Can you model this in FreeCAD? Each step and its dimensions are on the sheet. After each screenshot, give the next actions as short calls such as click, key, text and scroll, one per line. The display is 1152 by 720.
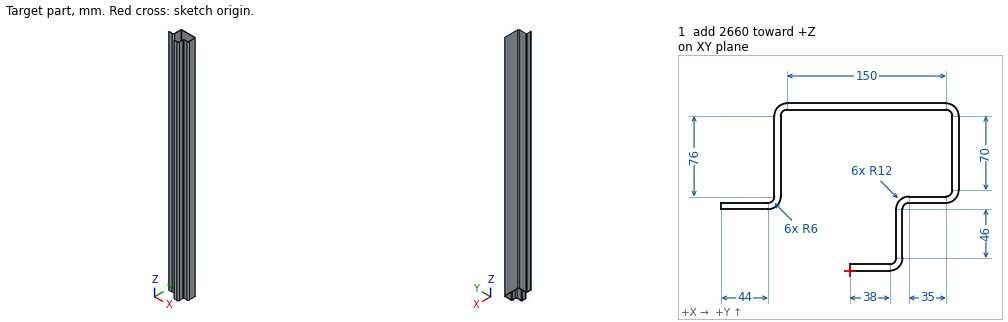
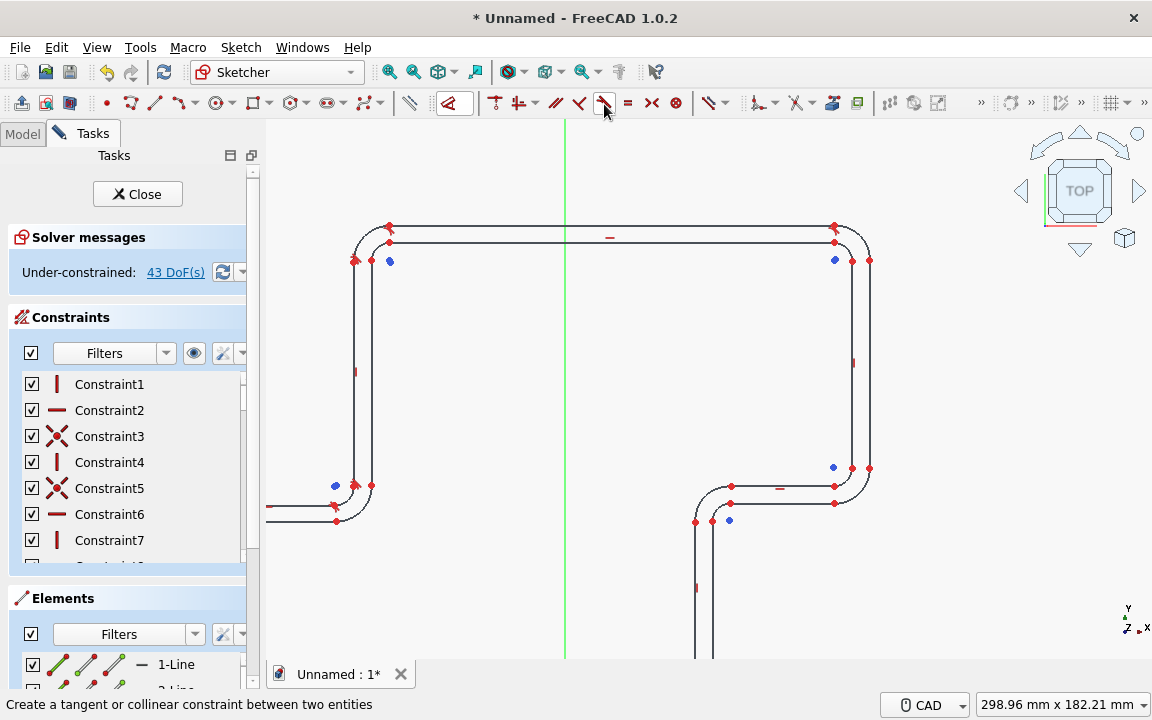
click(852, 323)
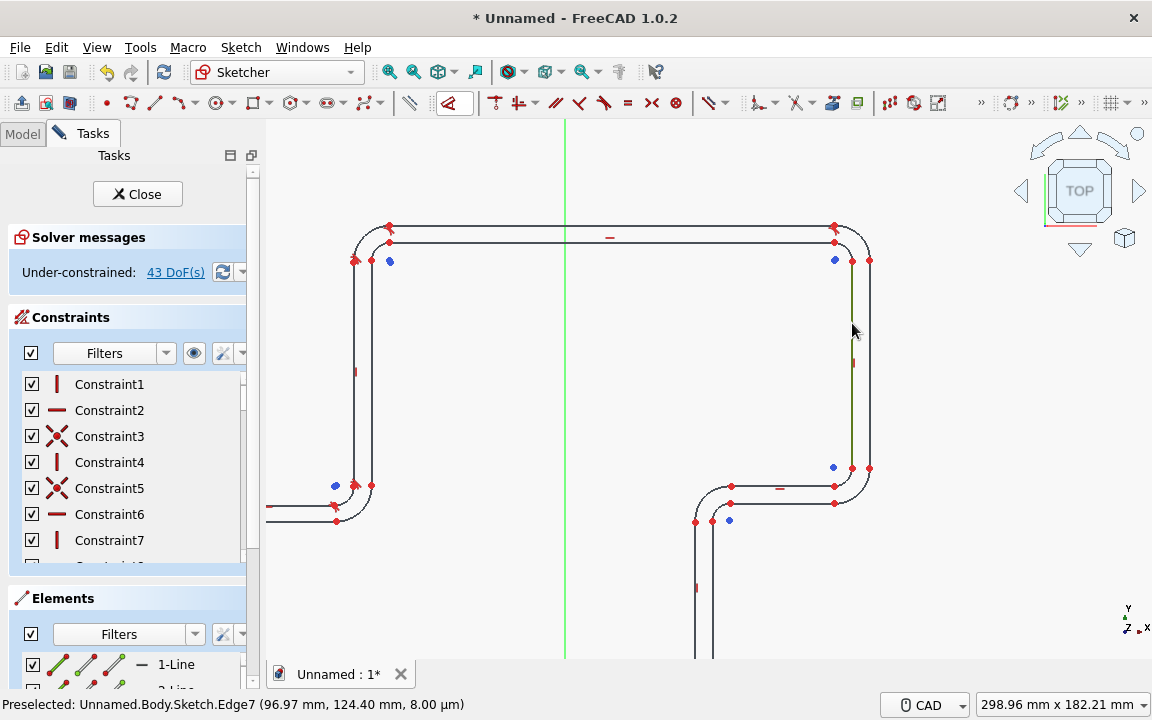
click(847, 248)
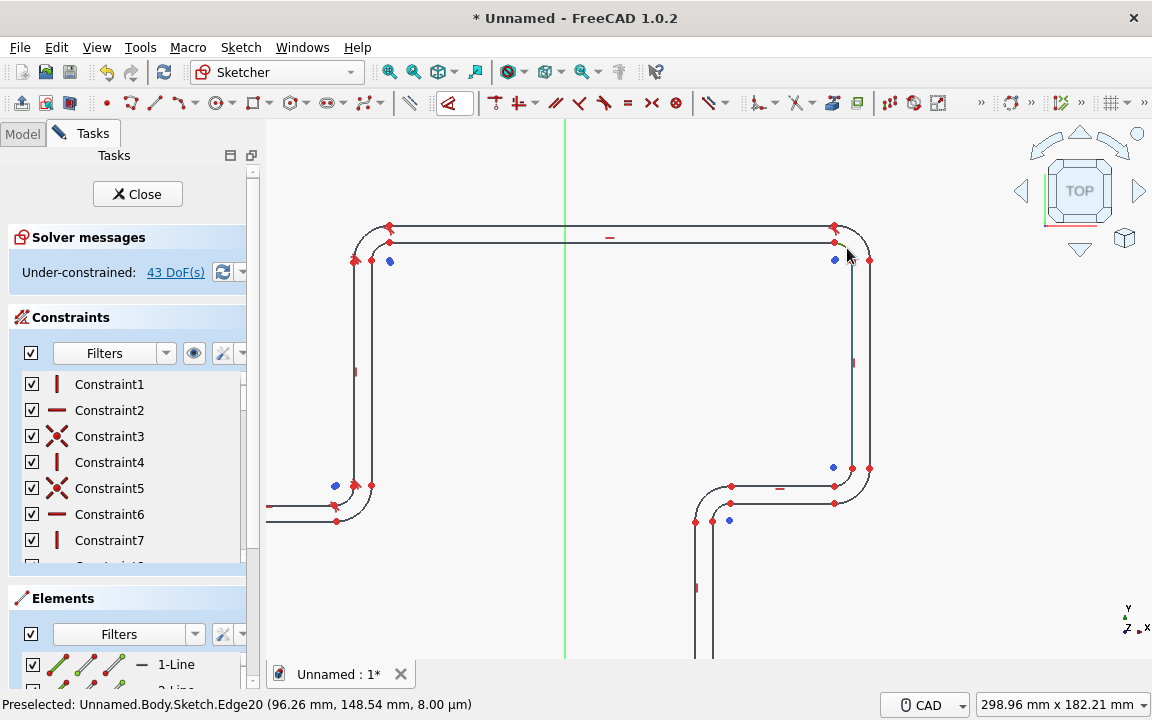
click(604, 104)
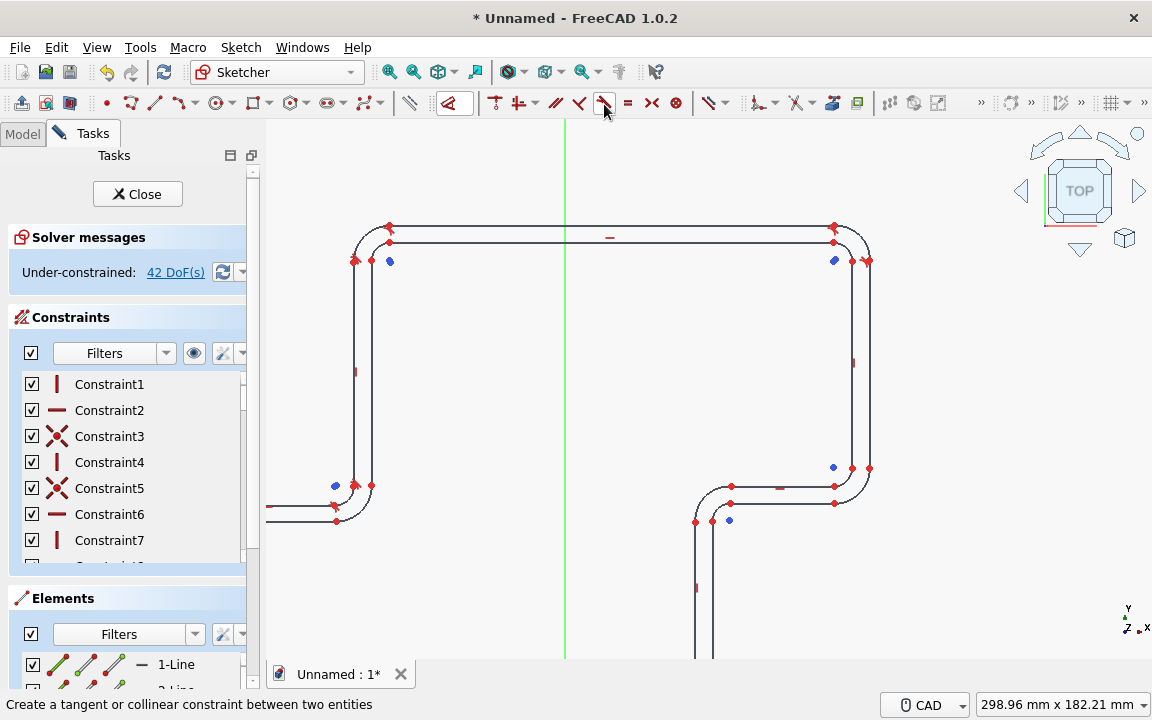
click(852, 323)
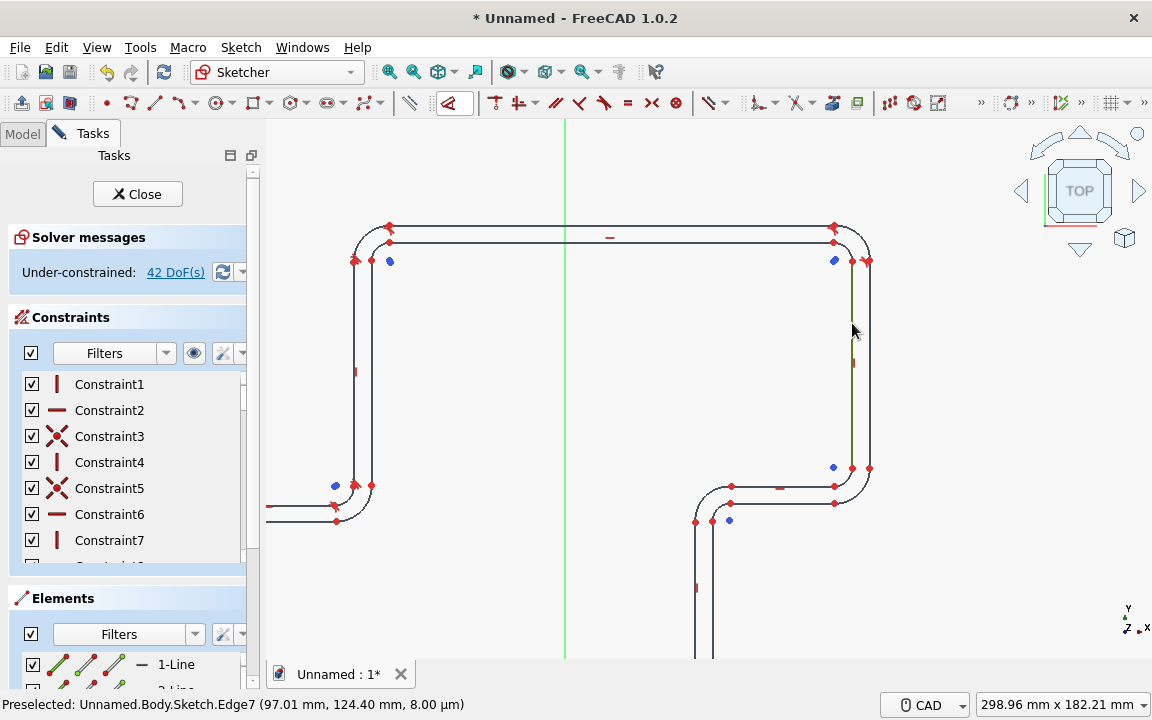
click(847, 481)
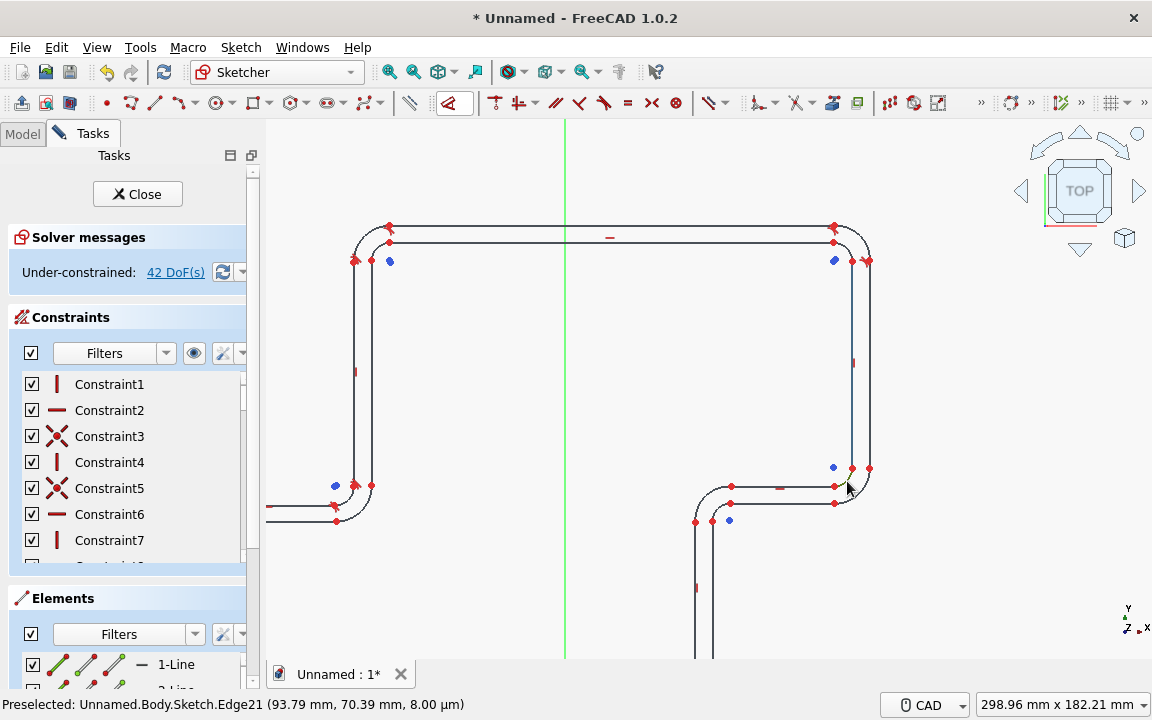
key(t)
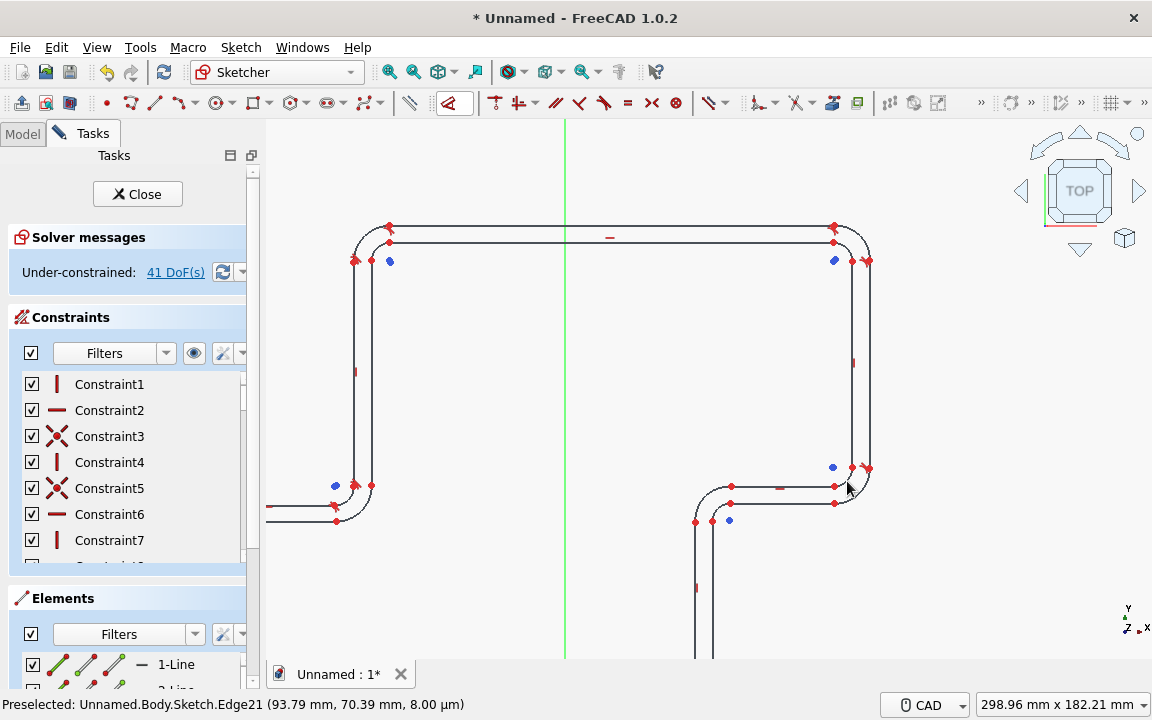
click(803, 487)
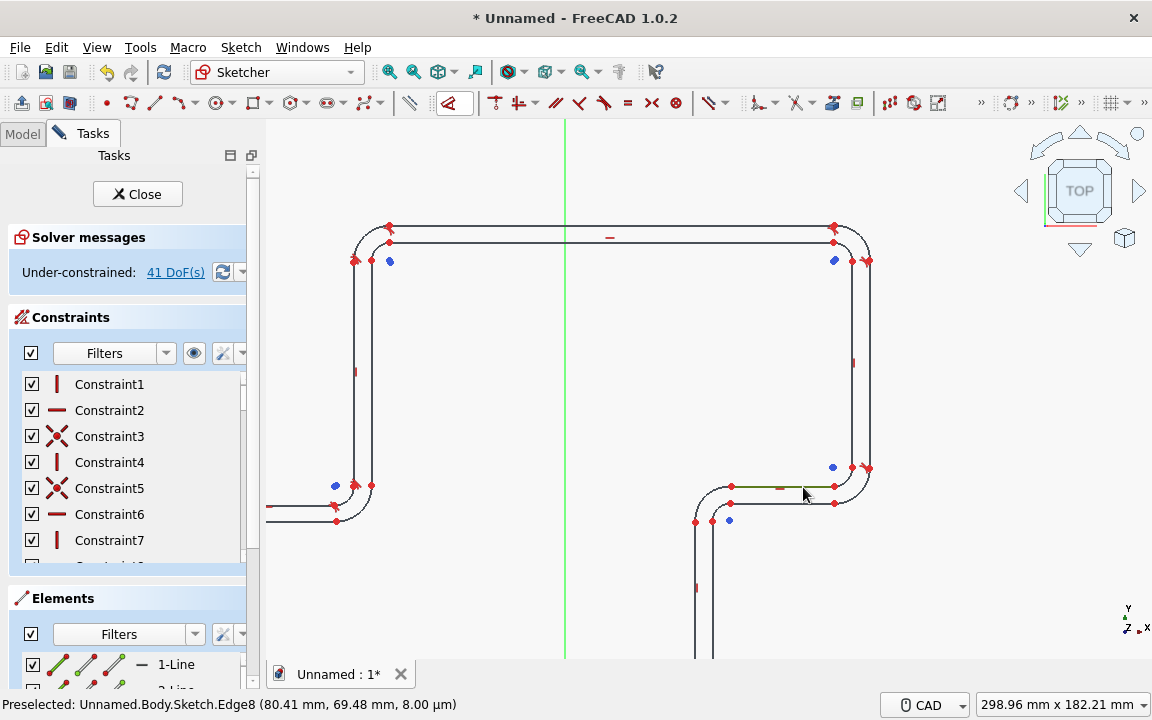
click(847, 481)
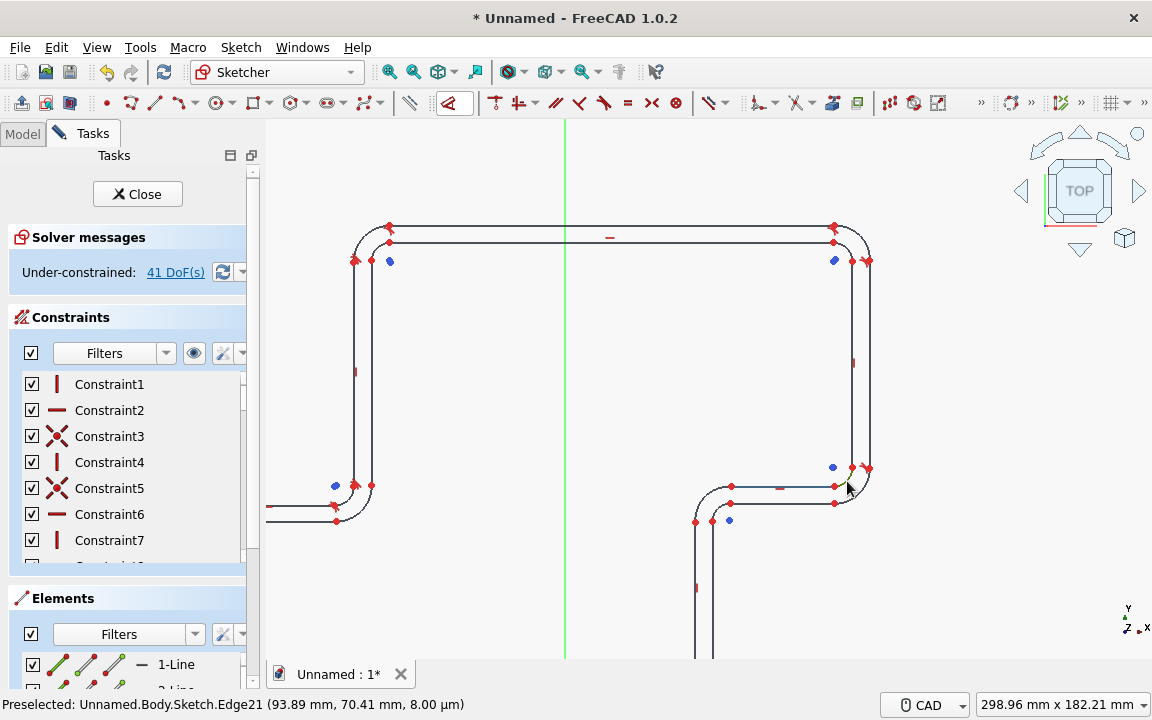
click(604, 104)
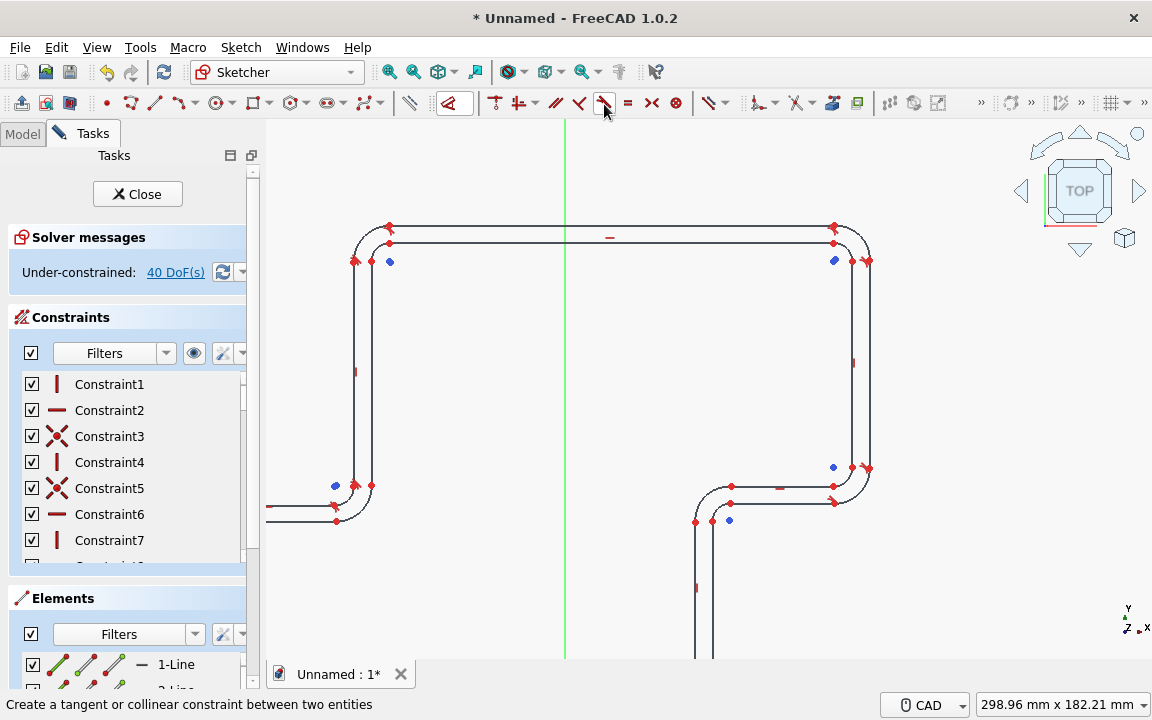
click(802, 487)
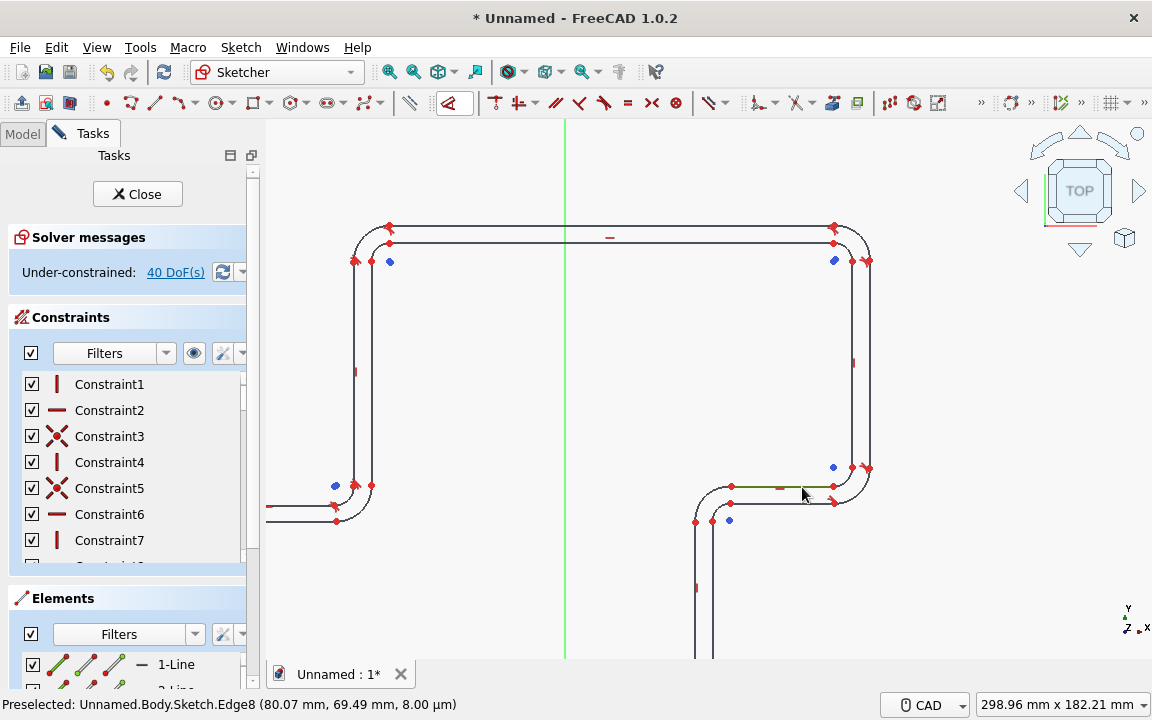
click(715, 490)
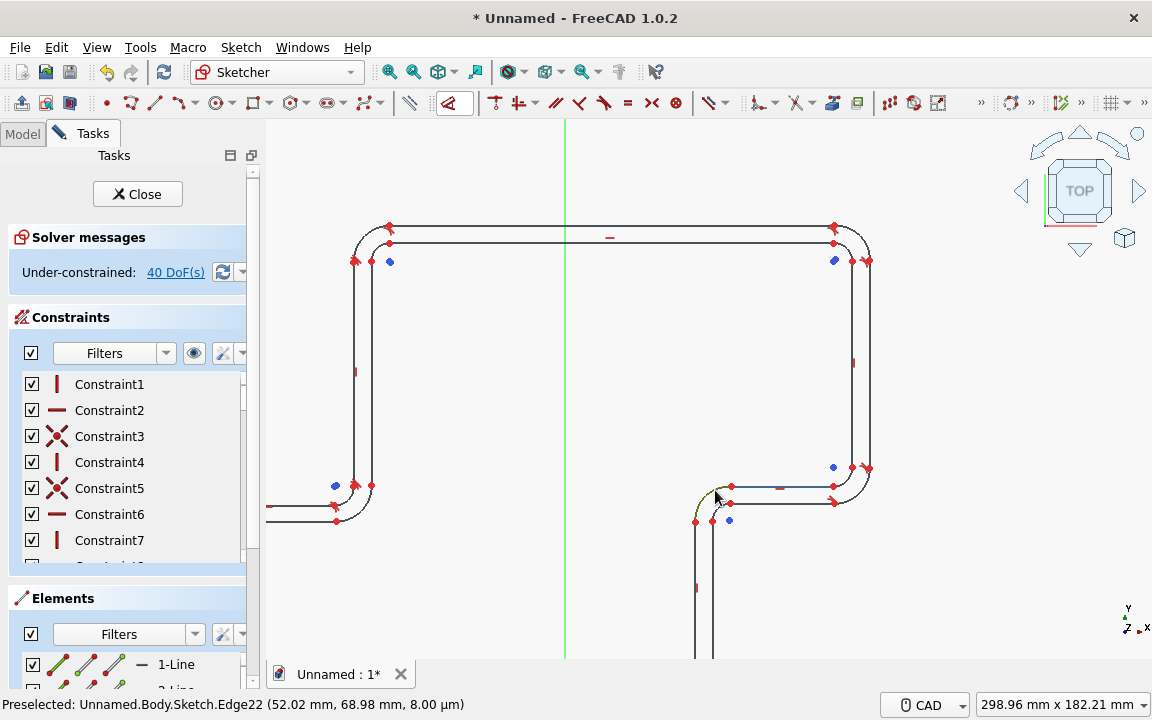
key(t)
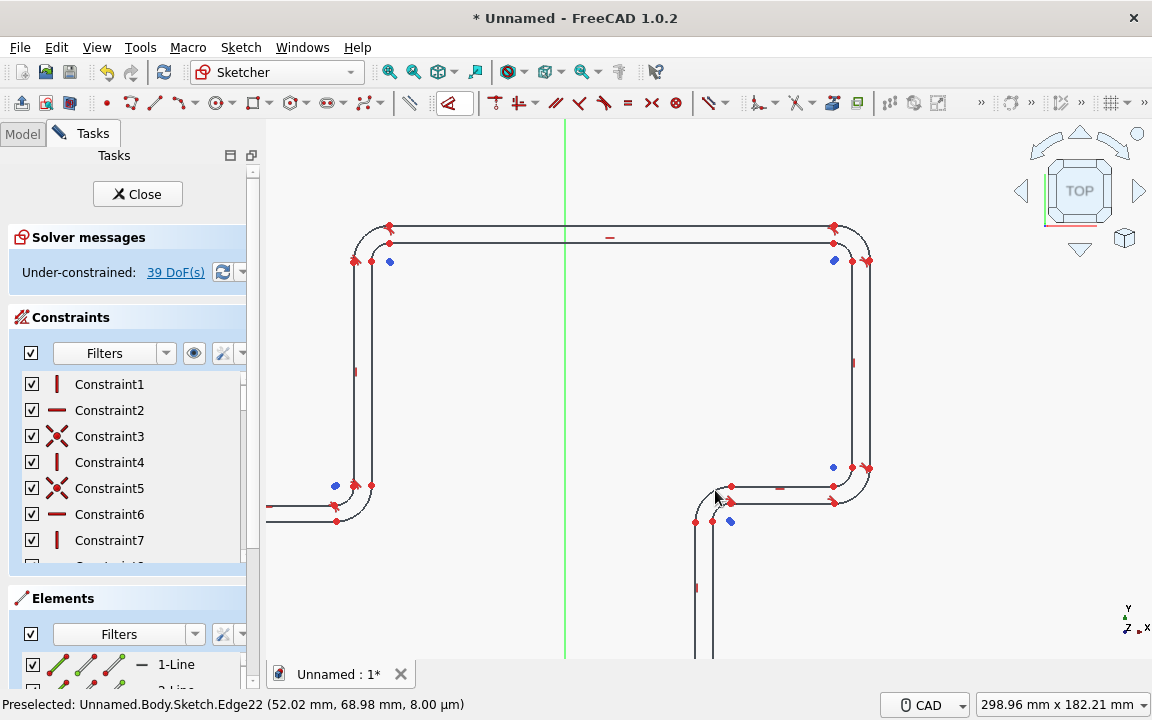
click(695, 563)